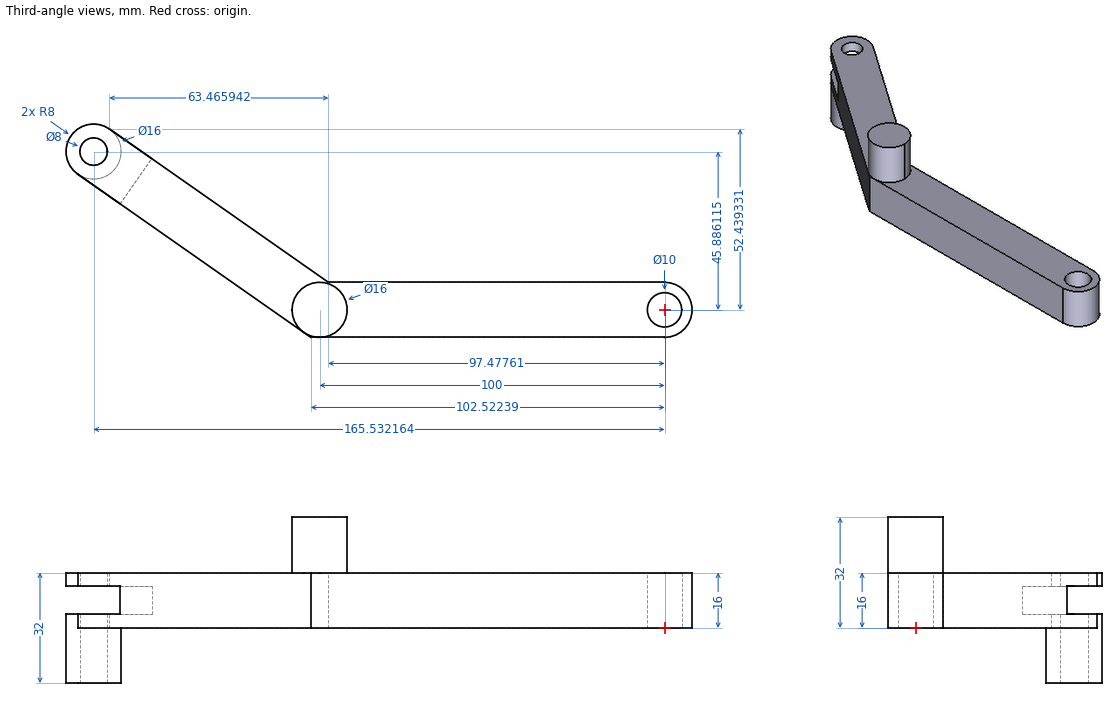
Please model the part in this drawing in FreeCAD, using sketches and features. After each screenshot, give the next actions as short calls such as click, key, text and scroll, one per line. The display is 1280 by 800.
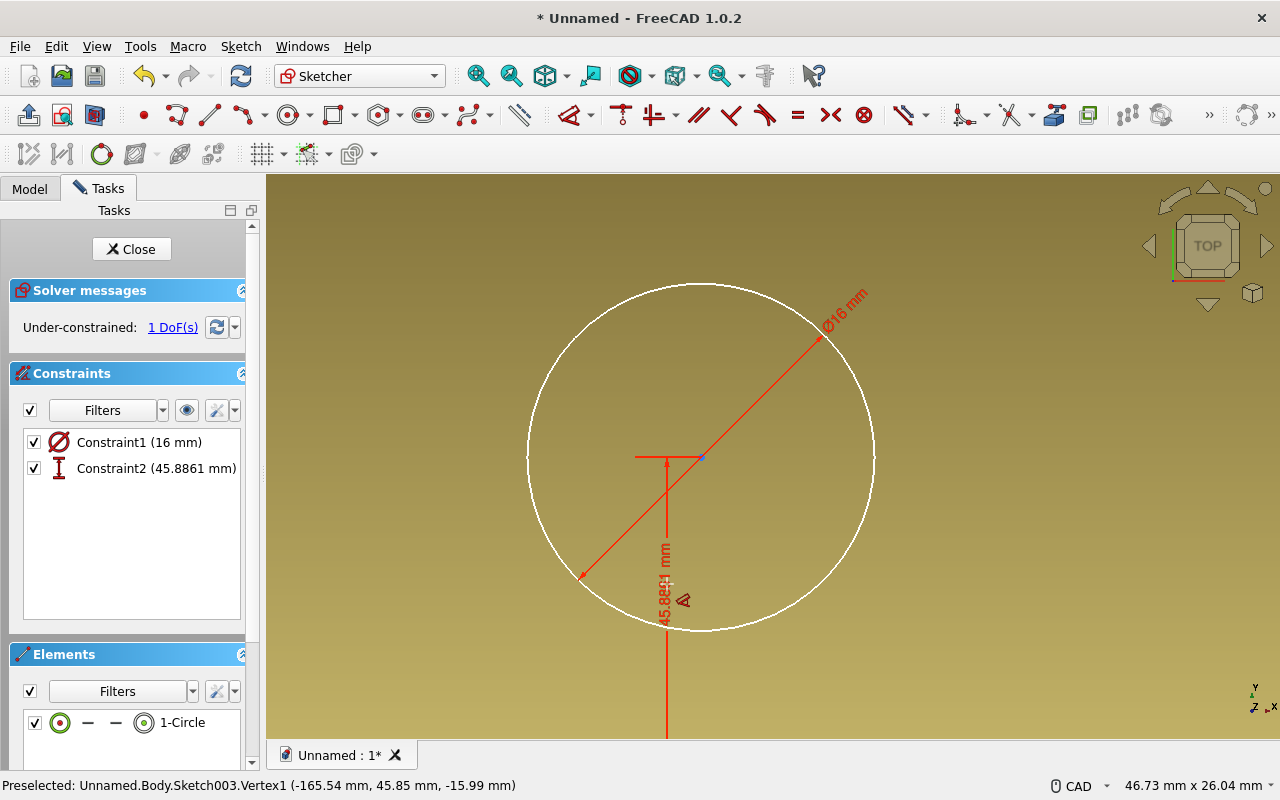
click(701, 457)
click(908, 423)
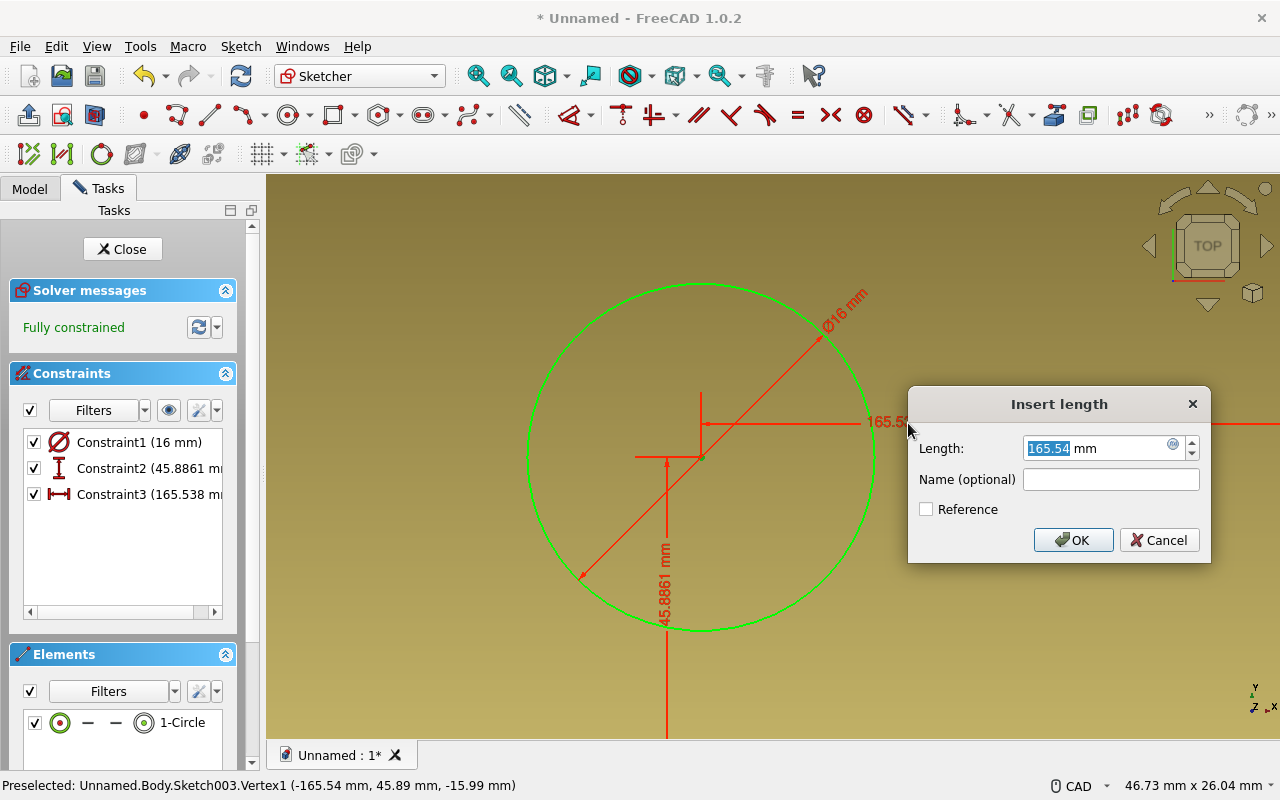
text(165.532164)
key(Return)
key(Escape)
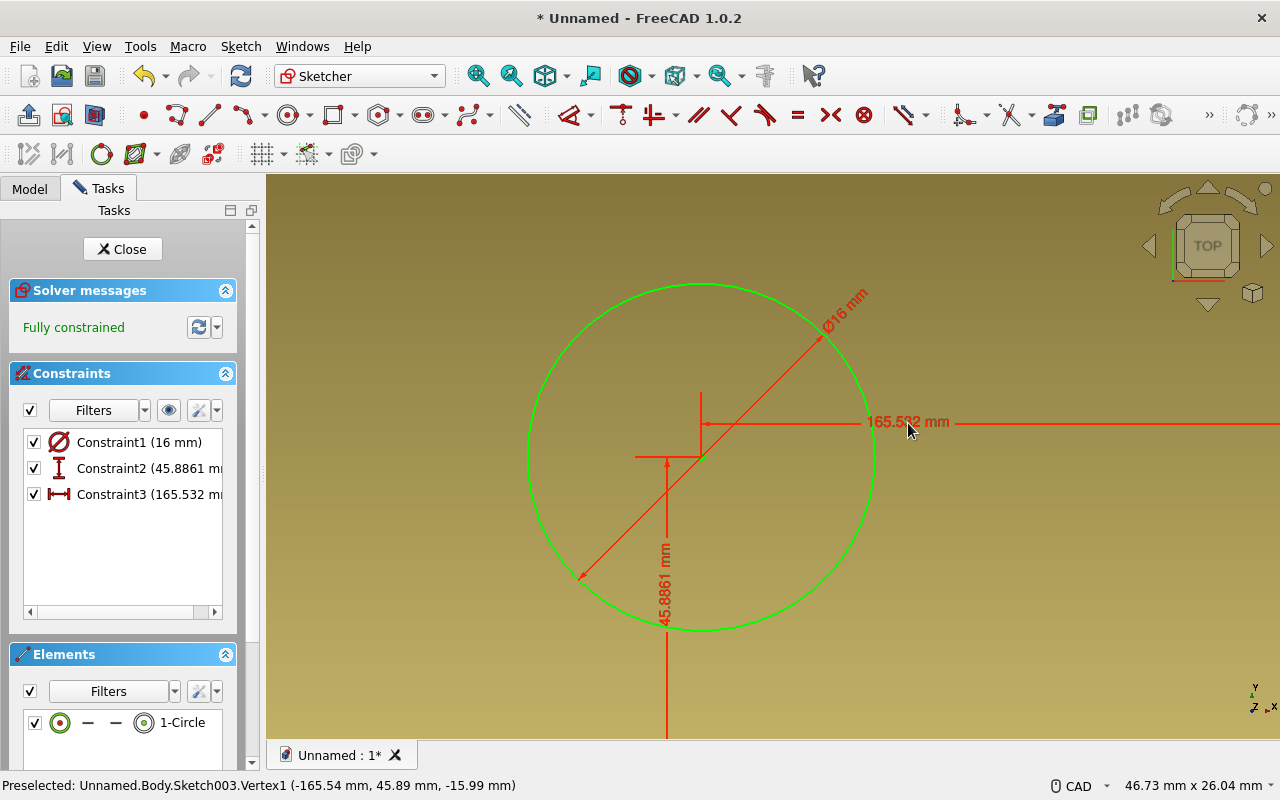
click(123, 249)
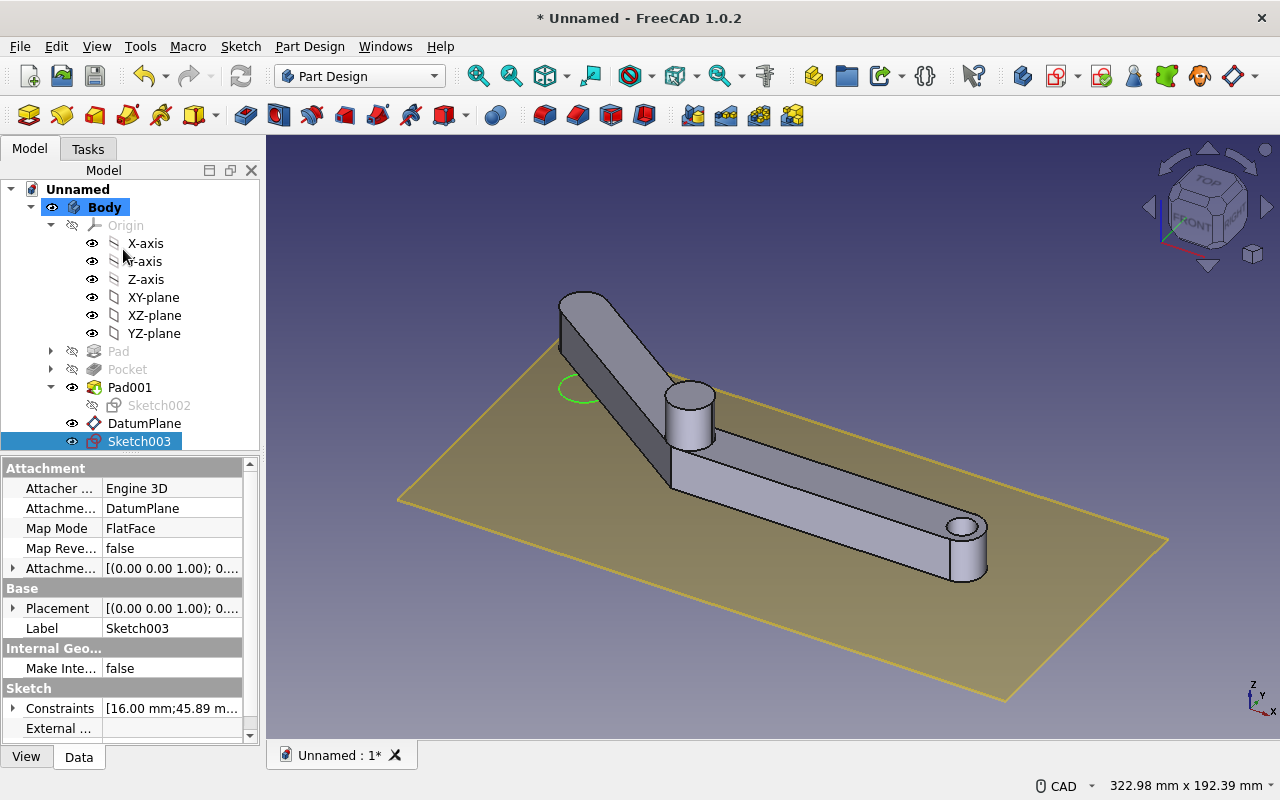
click(29, 116)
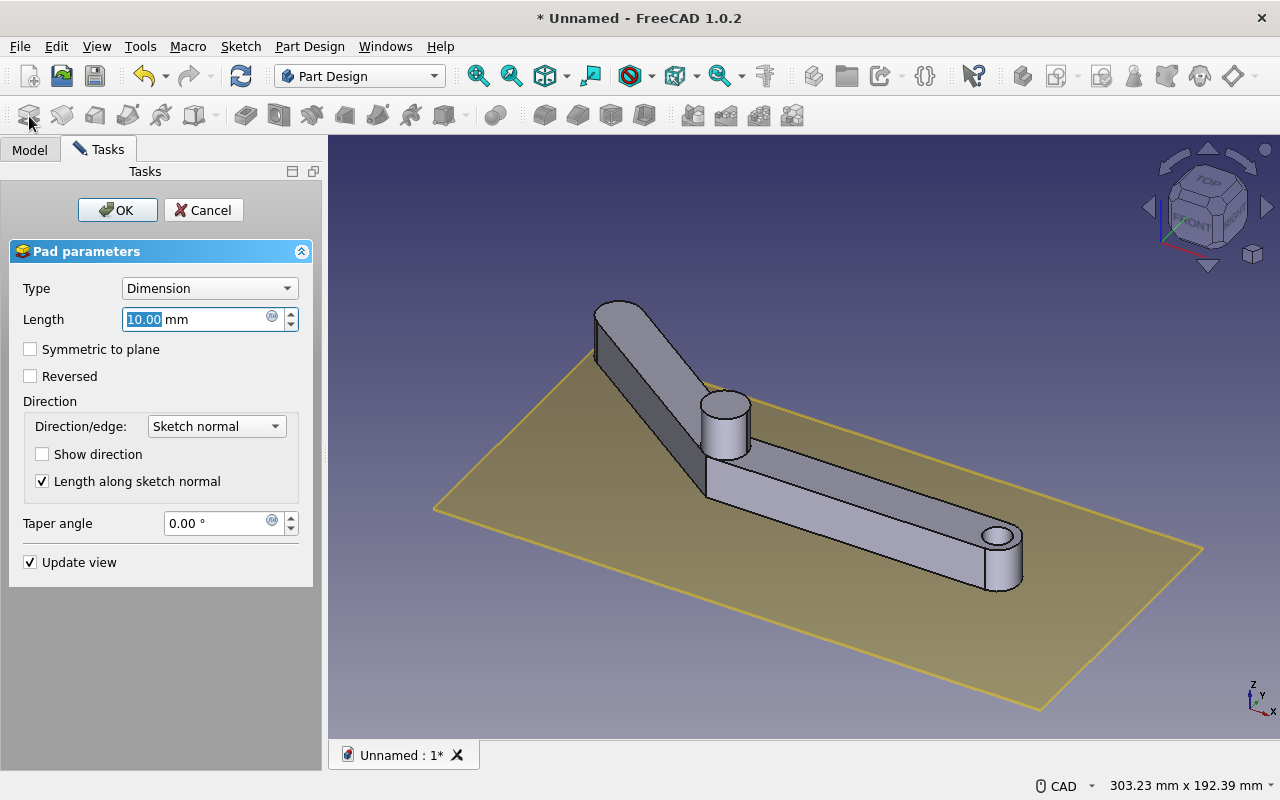
text(32)
key(Tab)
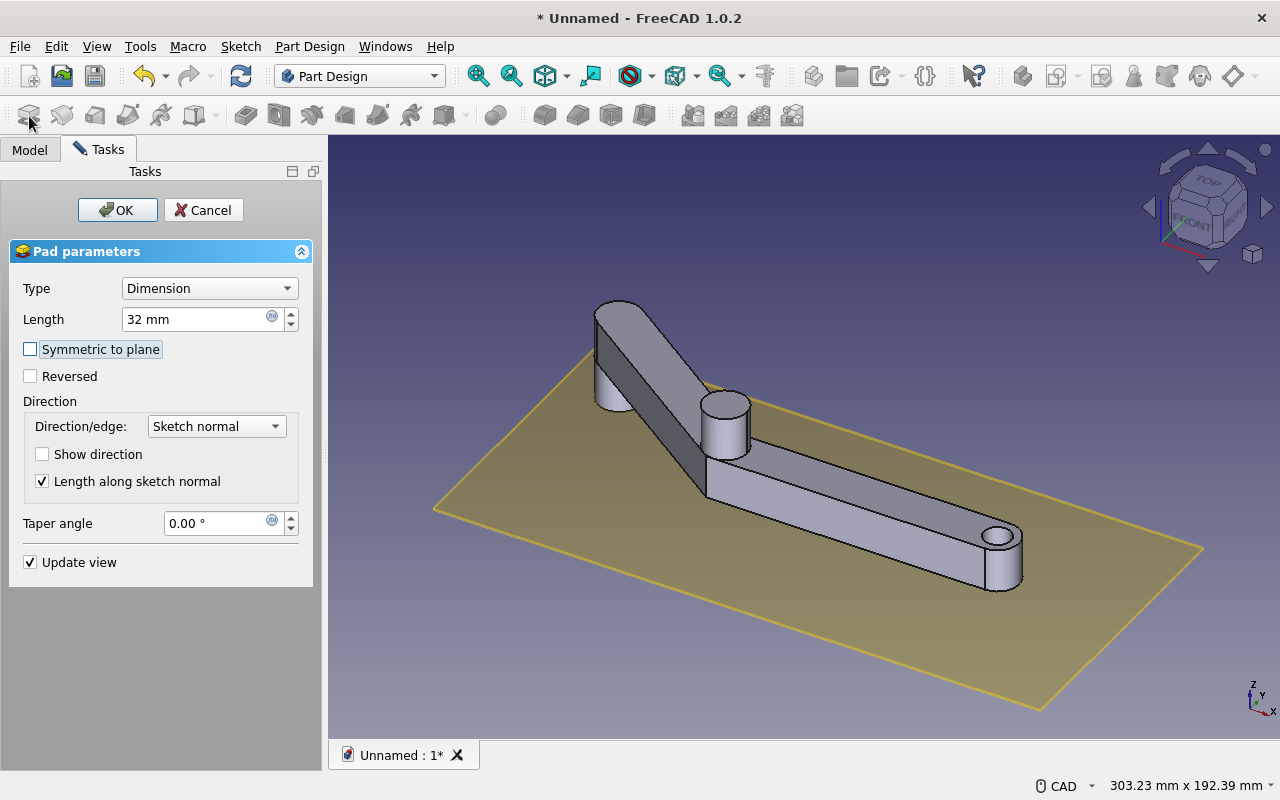
click(118, 210)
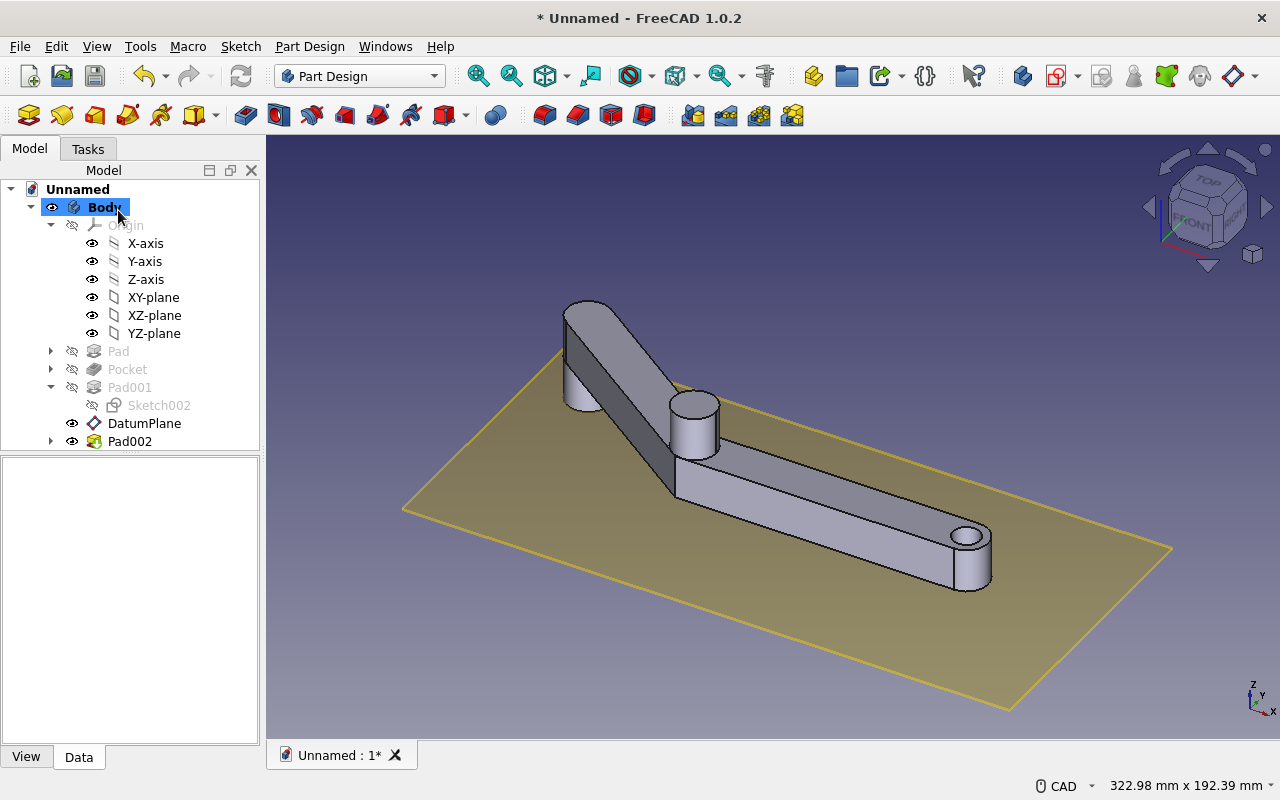
click(117, 423)
key(space)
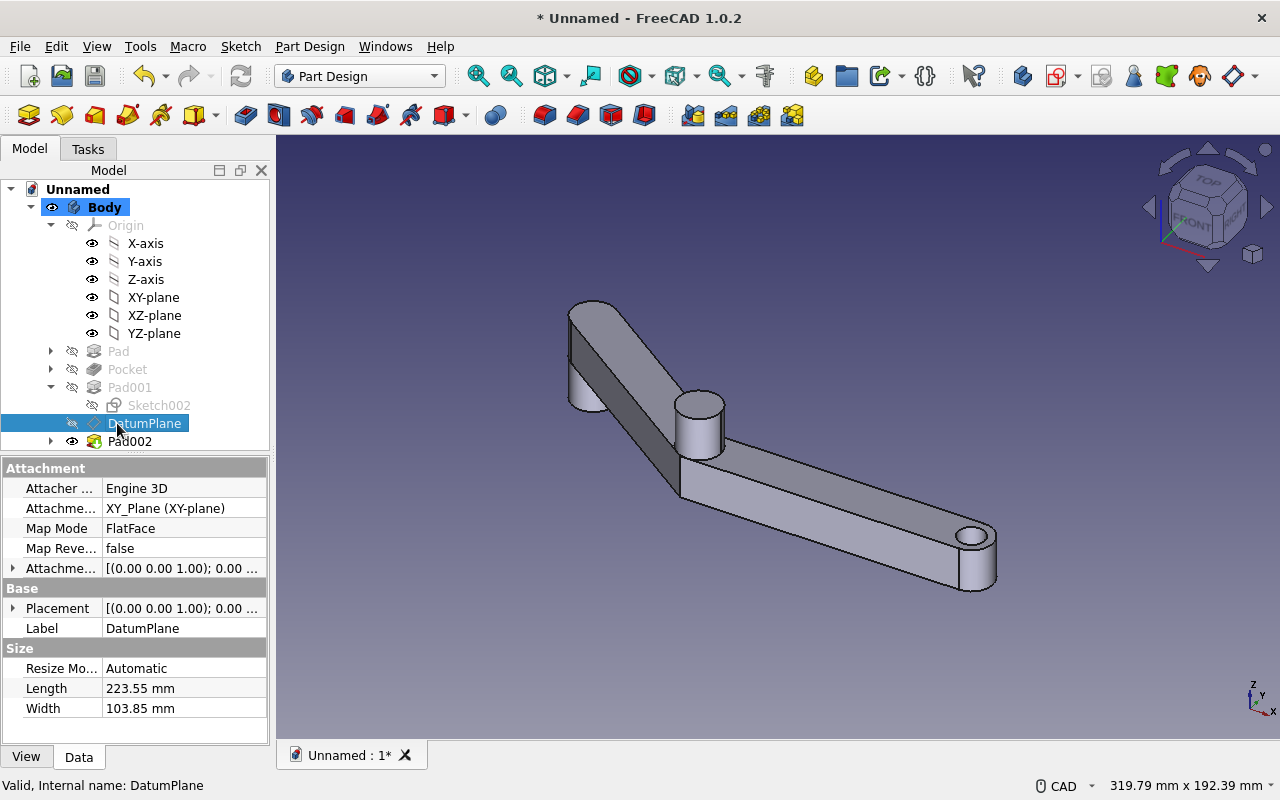
click(657, 447)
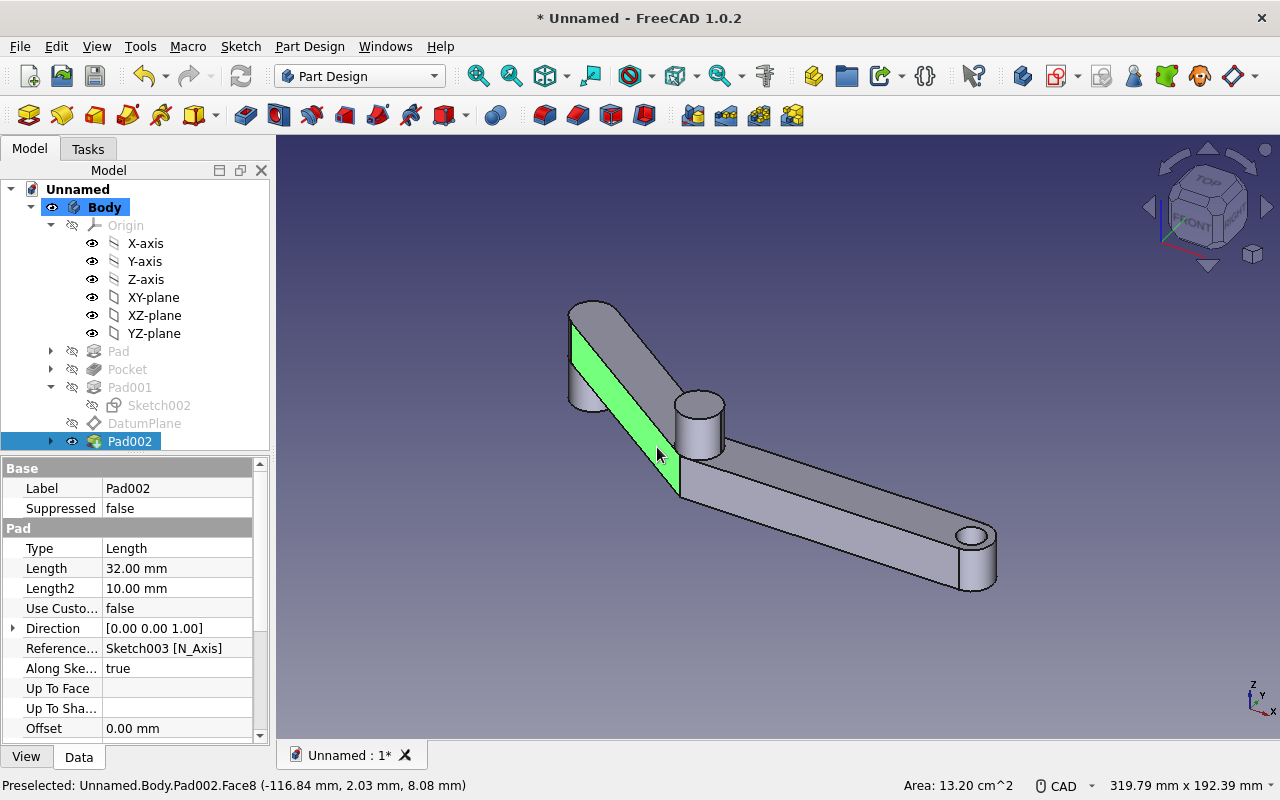
click(1056, 76)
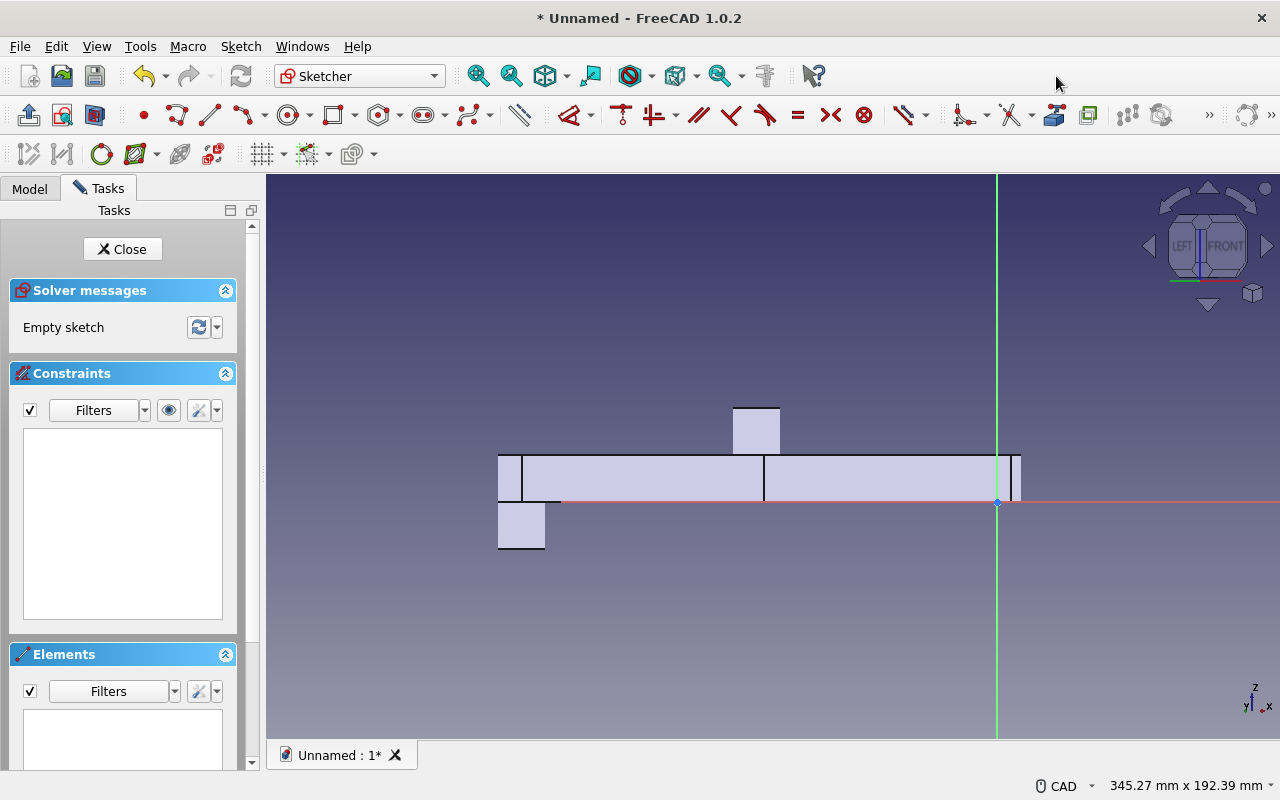
key(q)
key(s)